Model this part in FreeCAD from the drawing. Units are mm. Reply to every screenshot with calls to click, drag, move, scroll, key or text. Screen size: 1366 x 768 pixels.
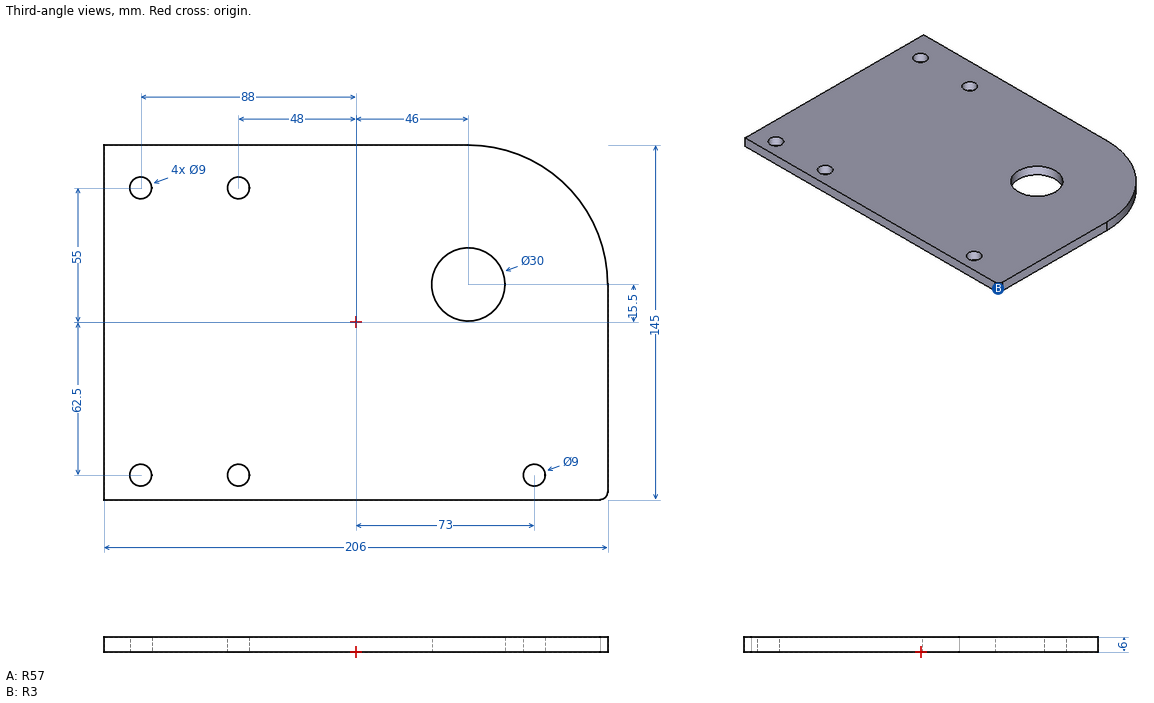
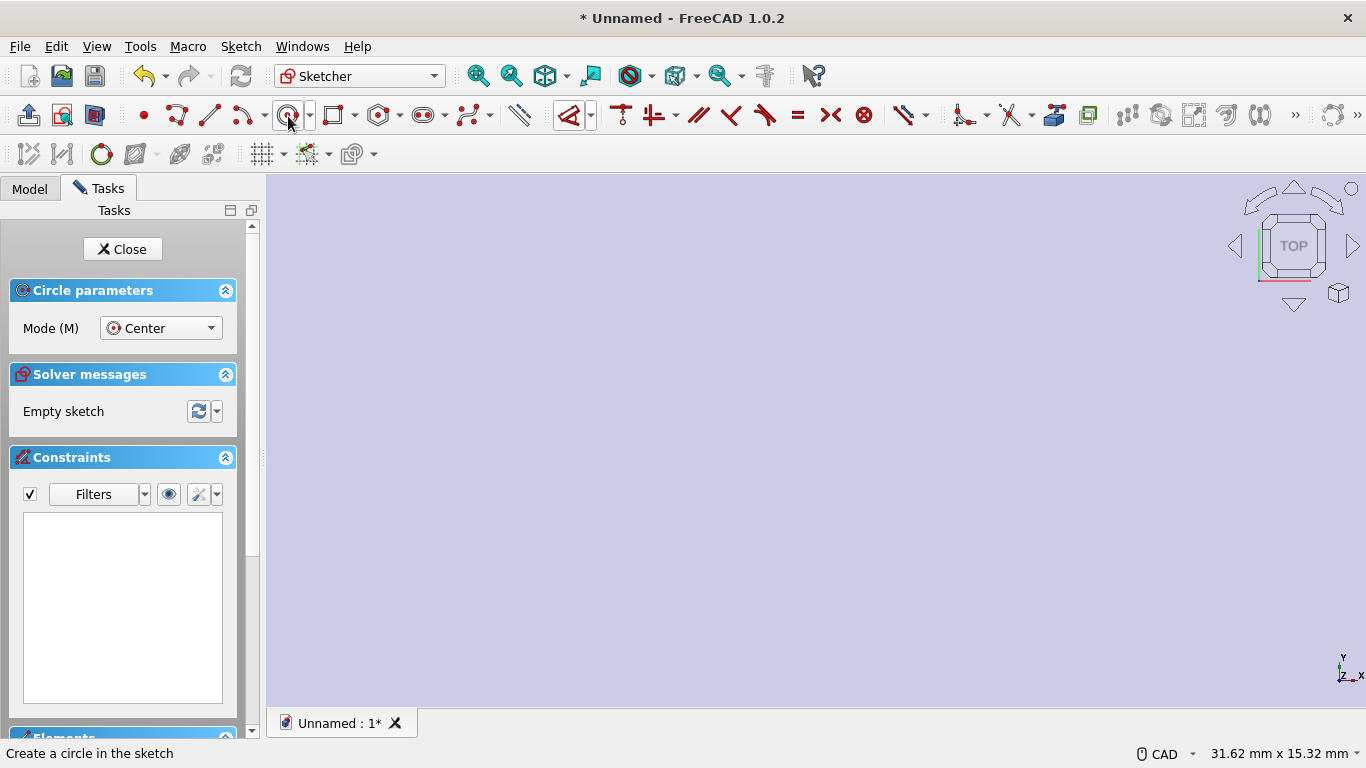
click(735, 433)
move(846, 322)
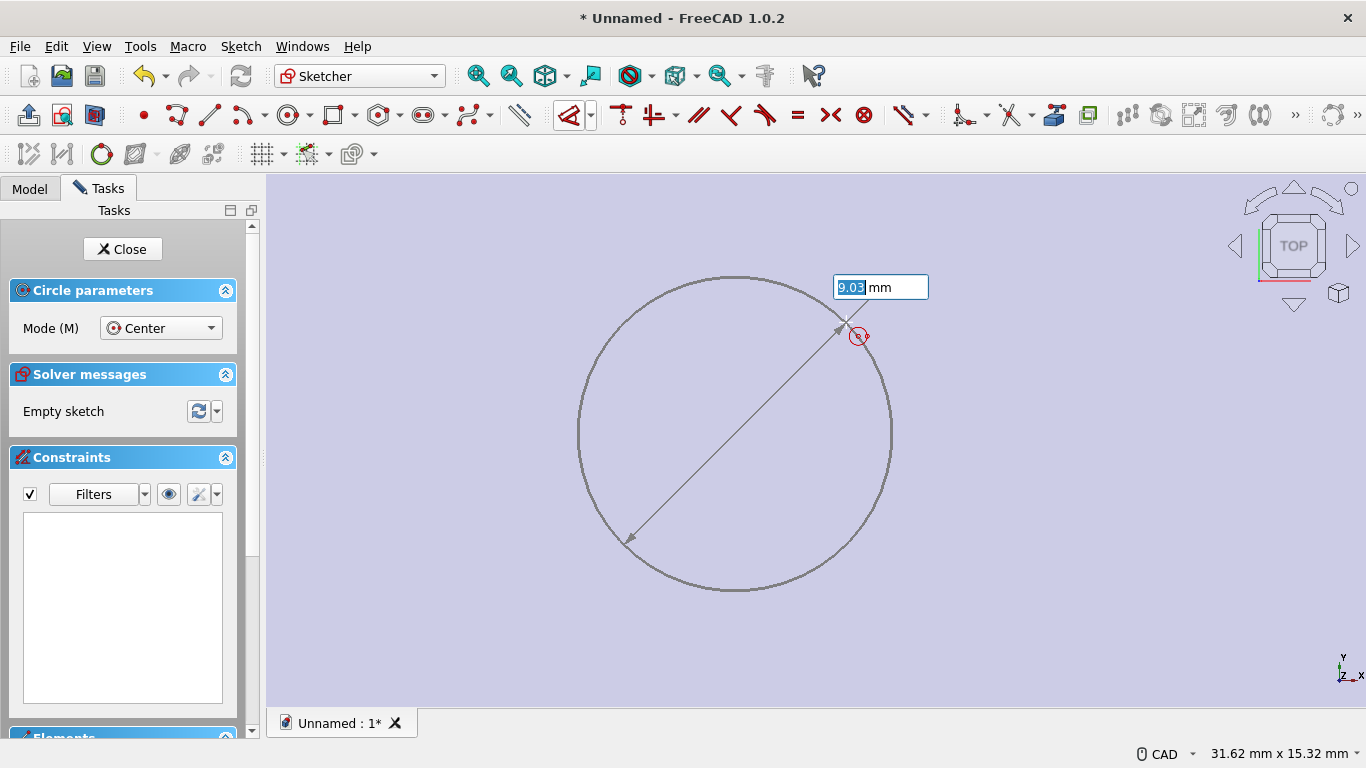
text(9)
key(Return)
key(Escape)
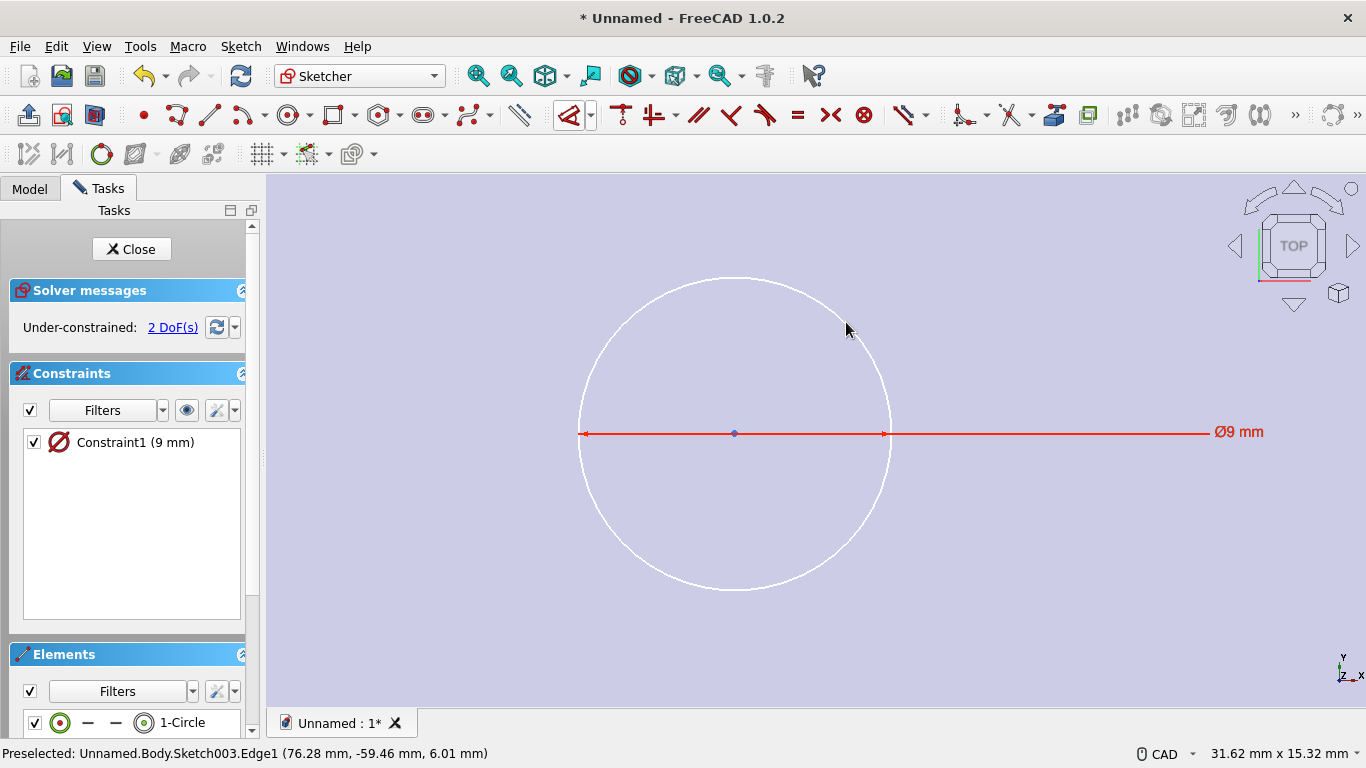
click(735, 434)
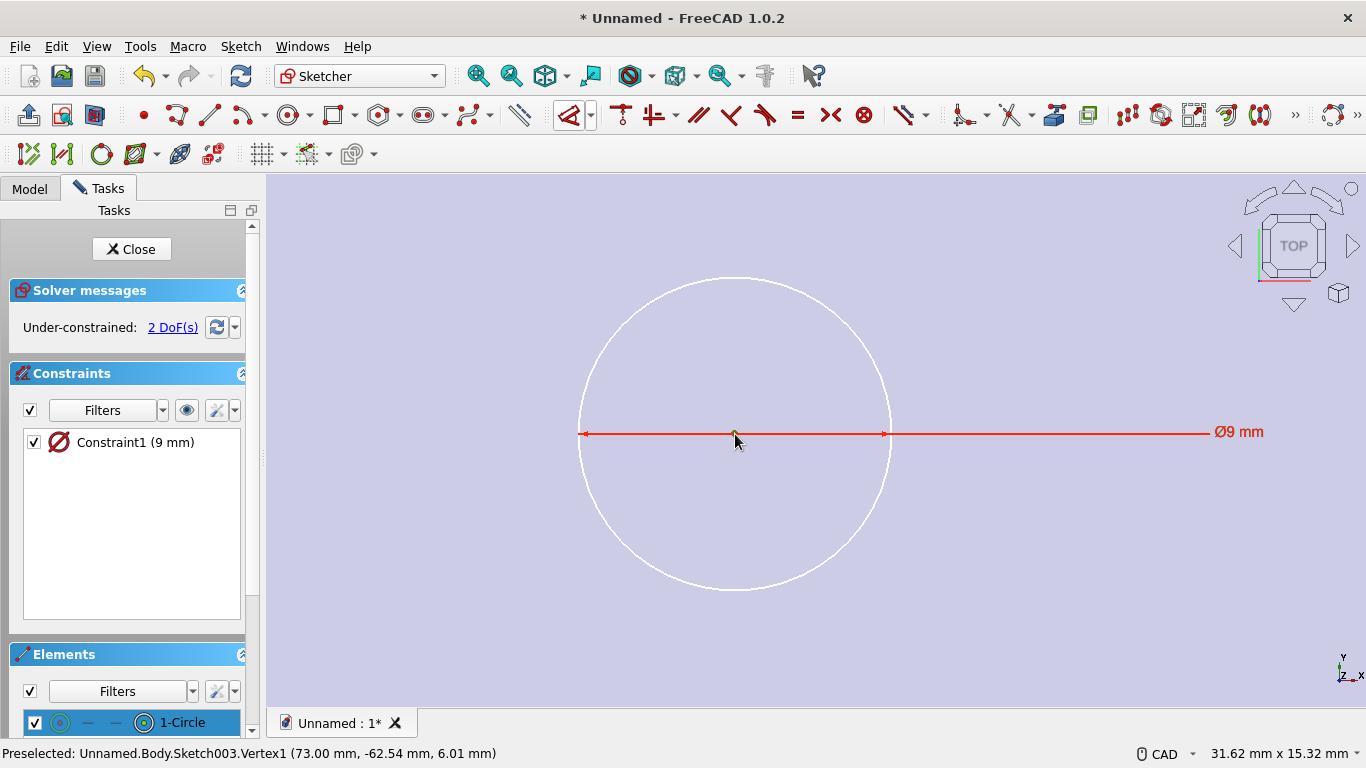
click(590, 116)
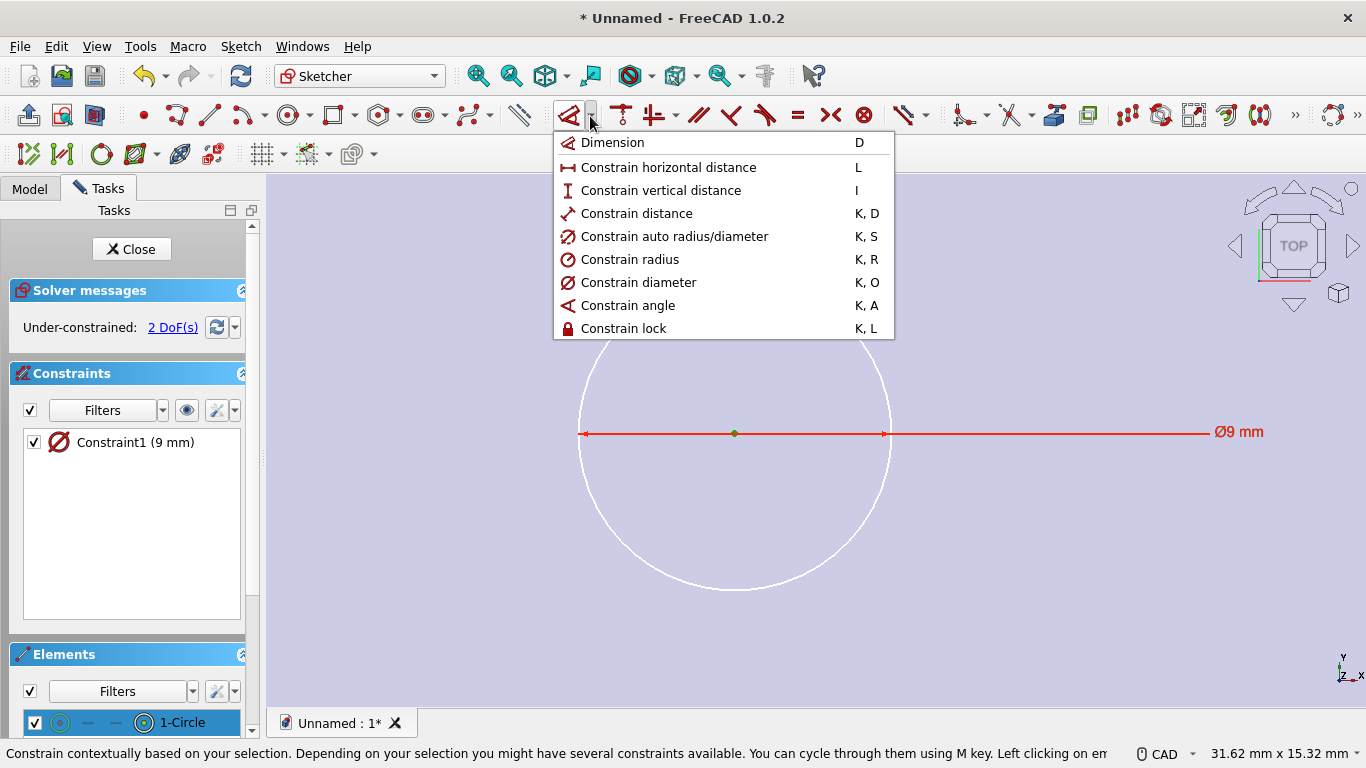
click(724, 168)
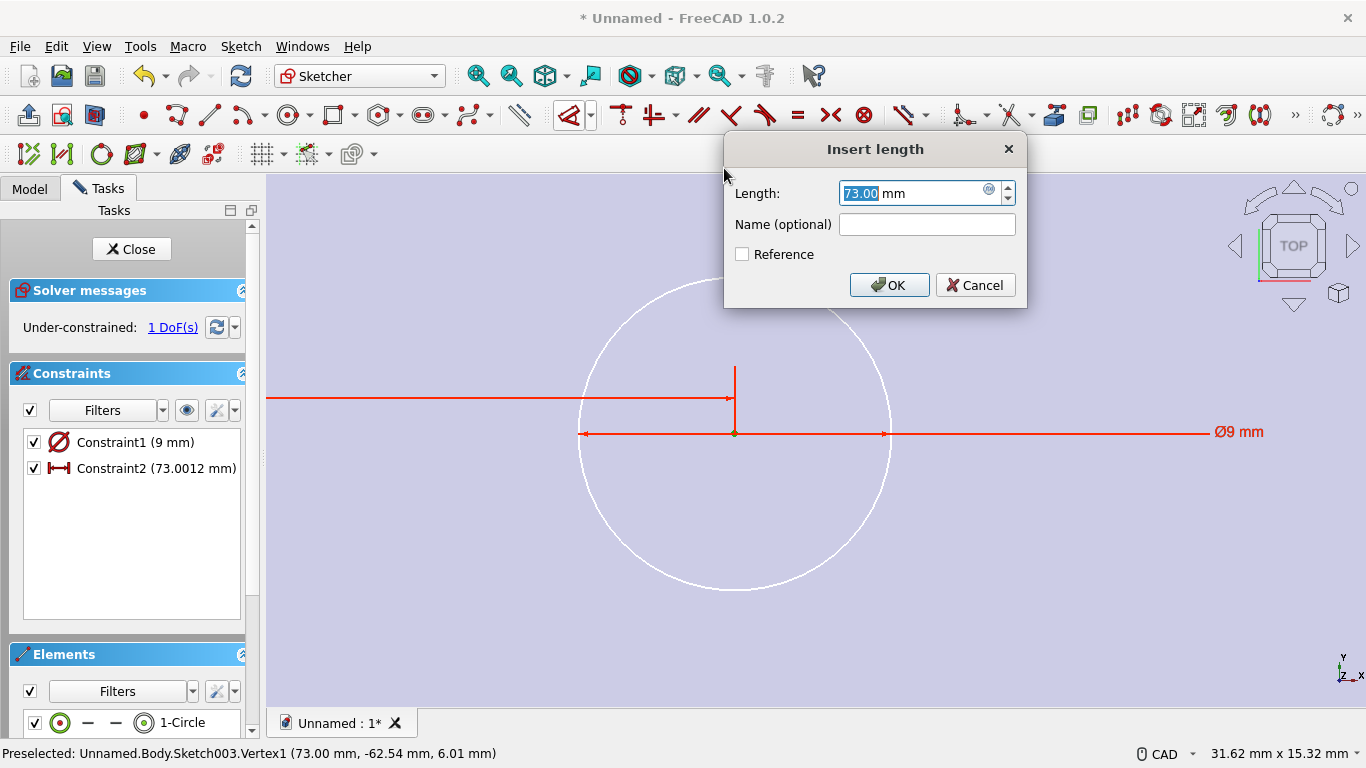
text(73)
key(Return)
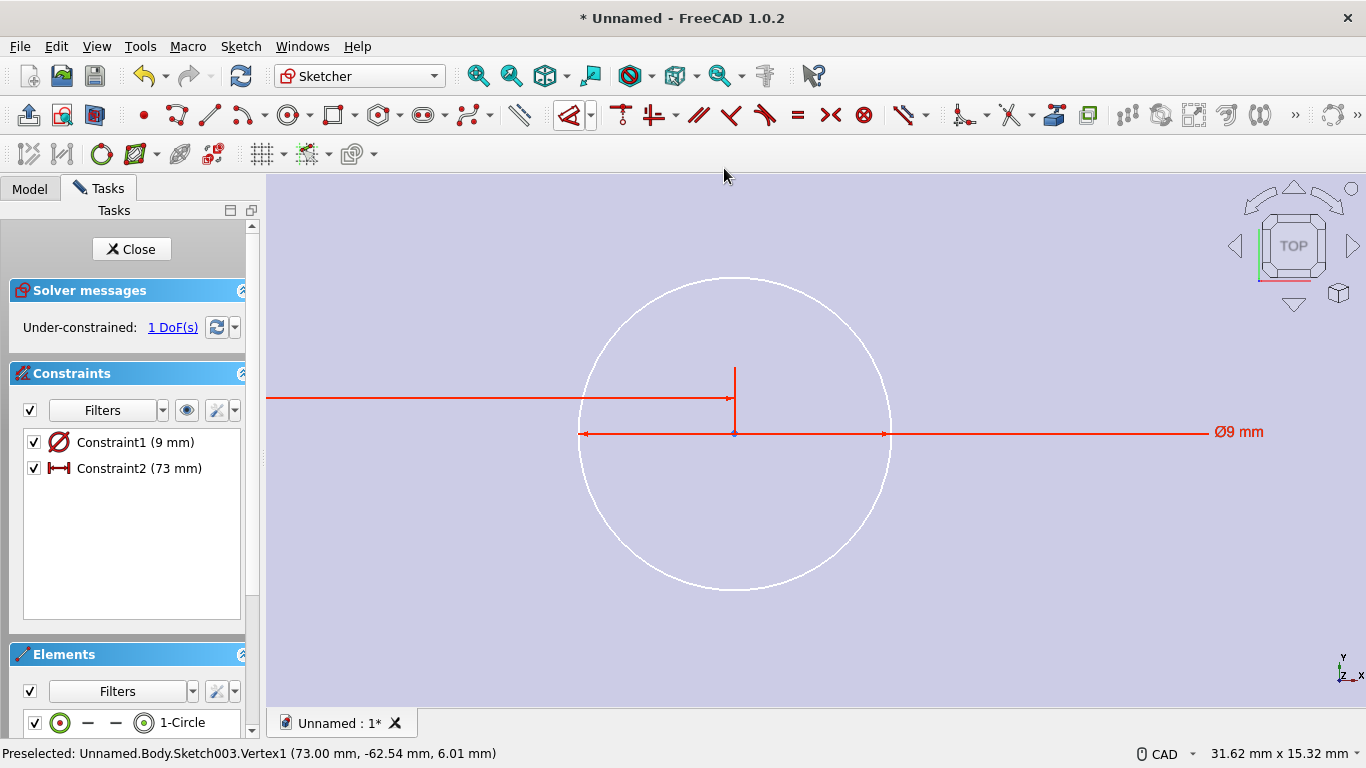
click(735, 434)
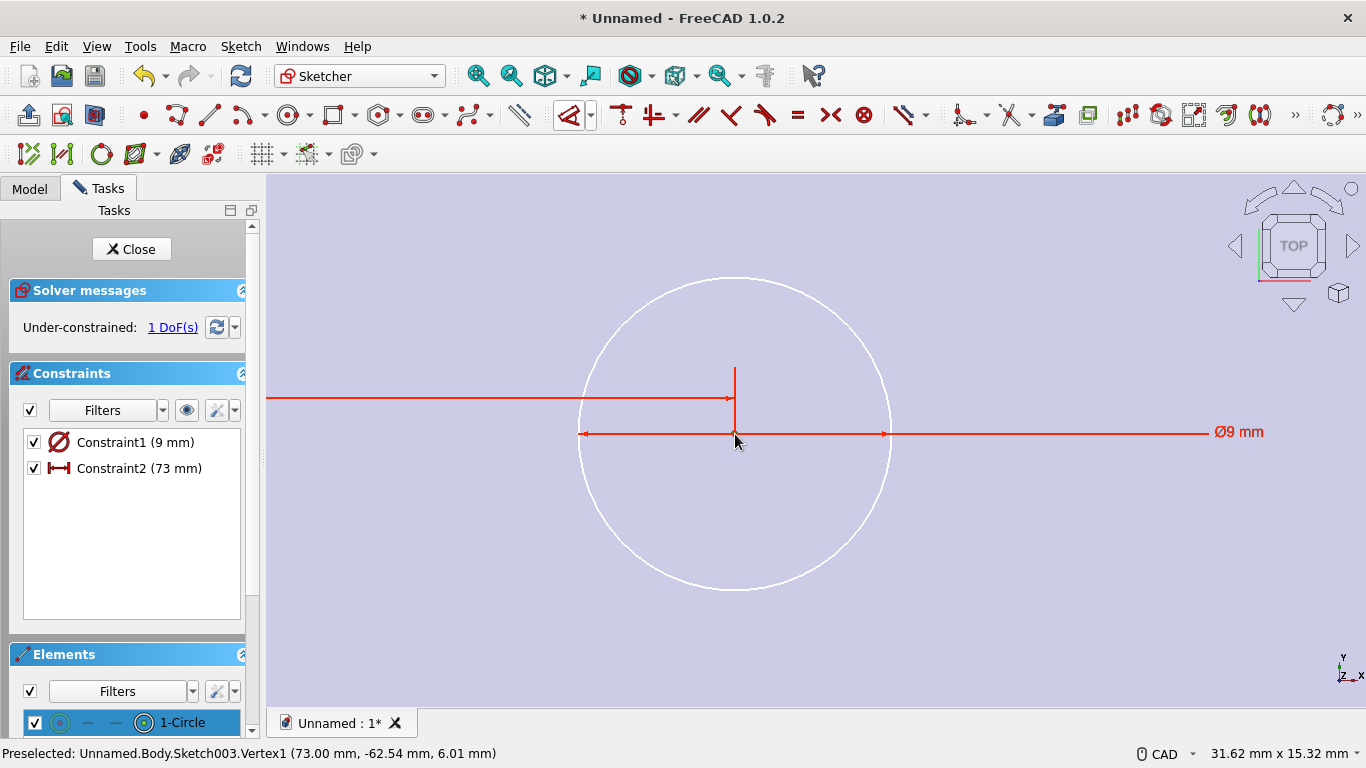
click(590, 116)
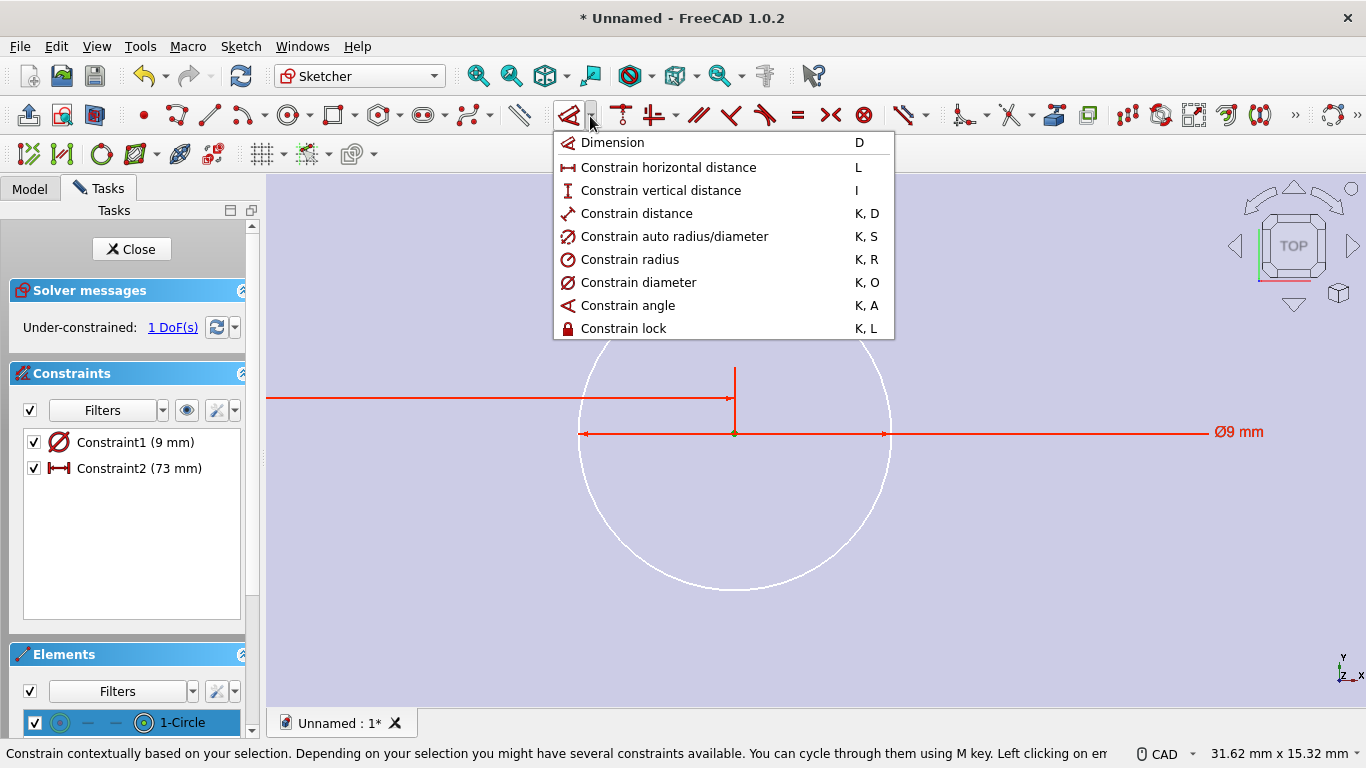
click(724, 190)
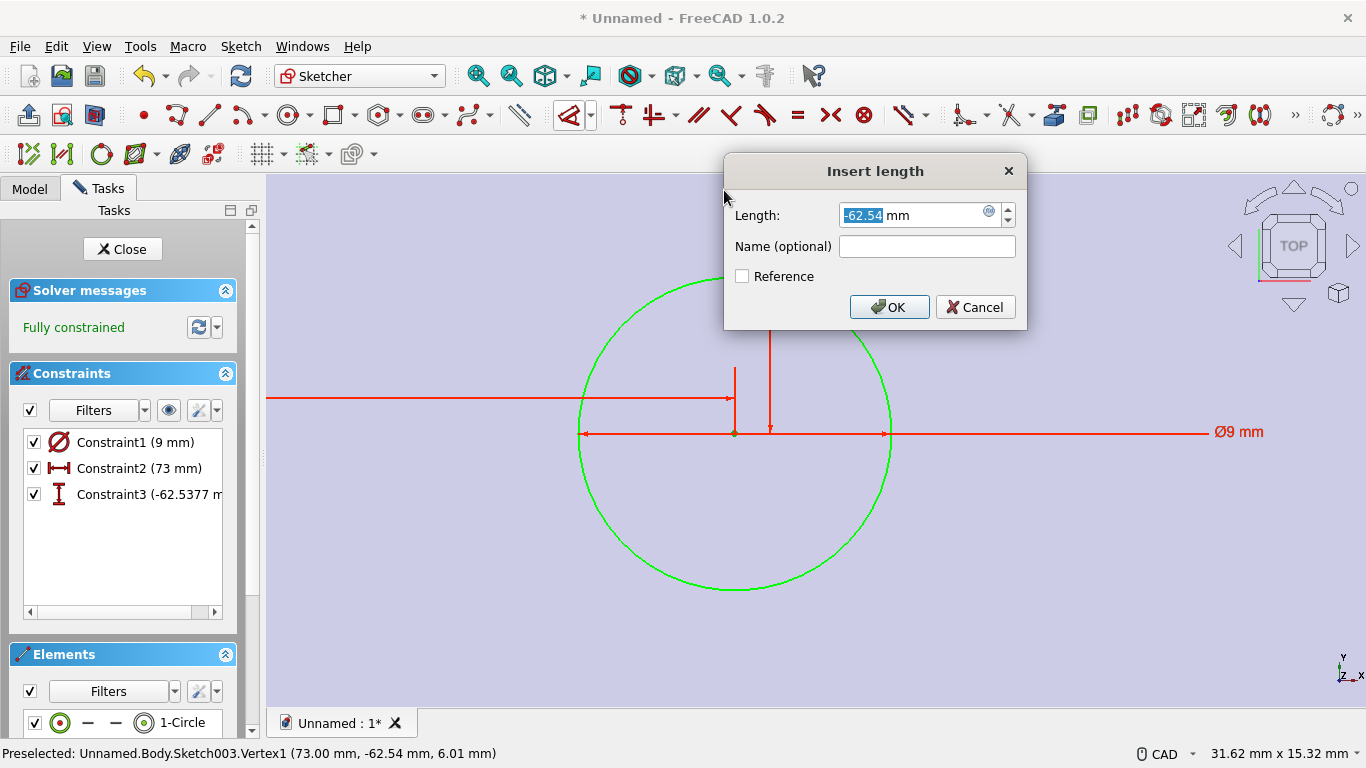
text(-62.5)
key(Return)